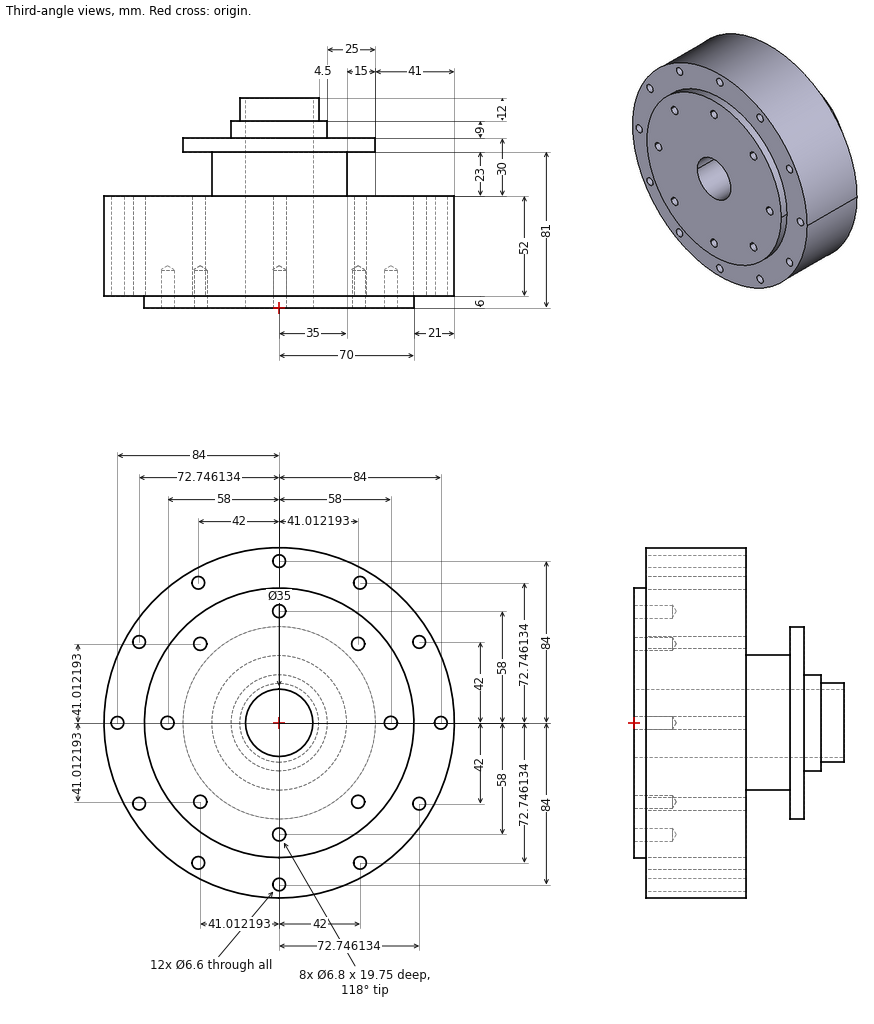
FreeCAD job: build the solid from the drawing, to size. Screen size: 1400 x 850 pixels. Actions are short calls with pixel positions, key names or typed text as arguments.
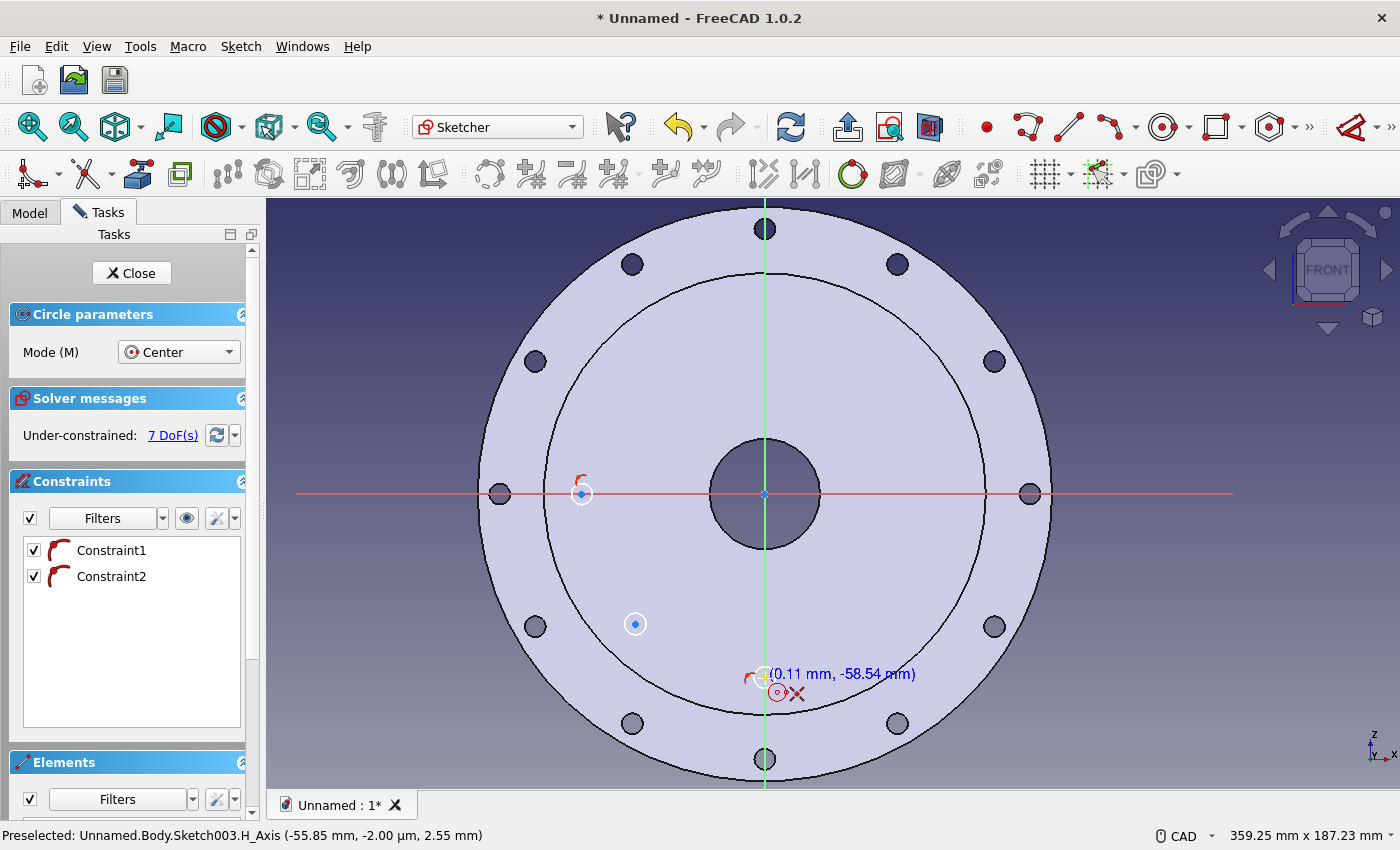
scroll(635, 365, up, 4)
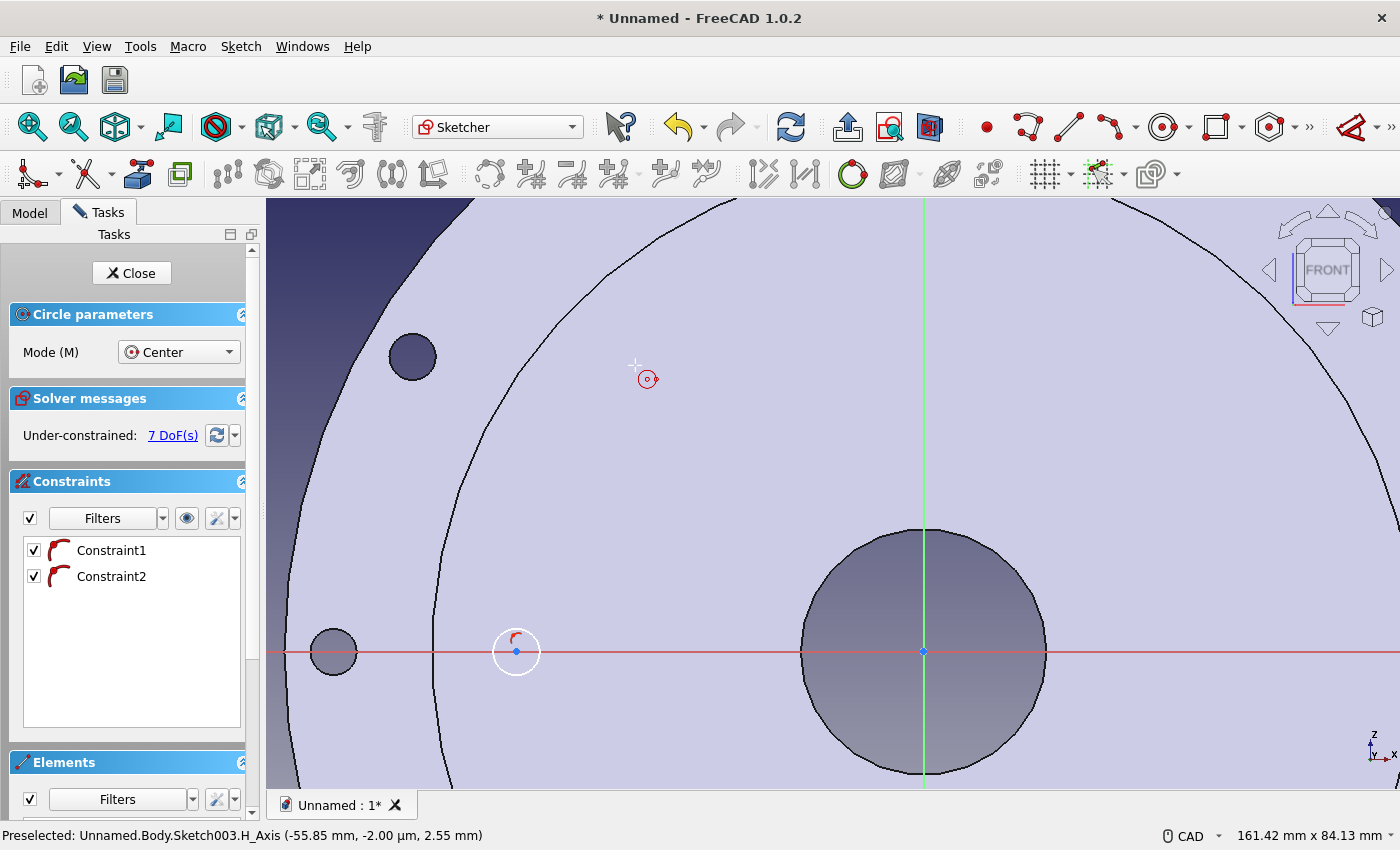
click(636, 364)
click(652, 347)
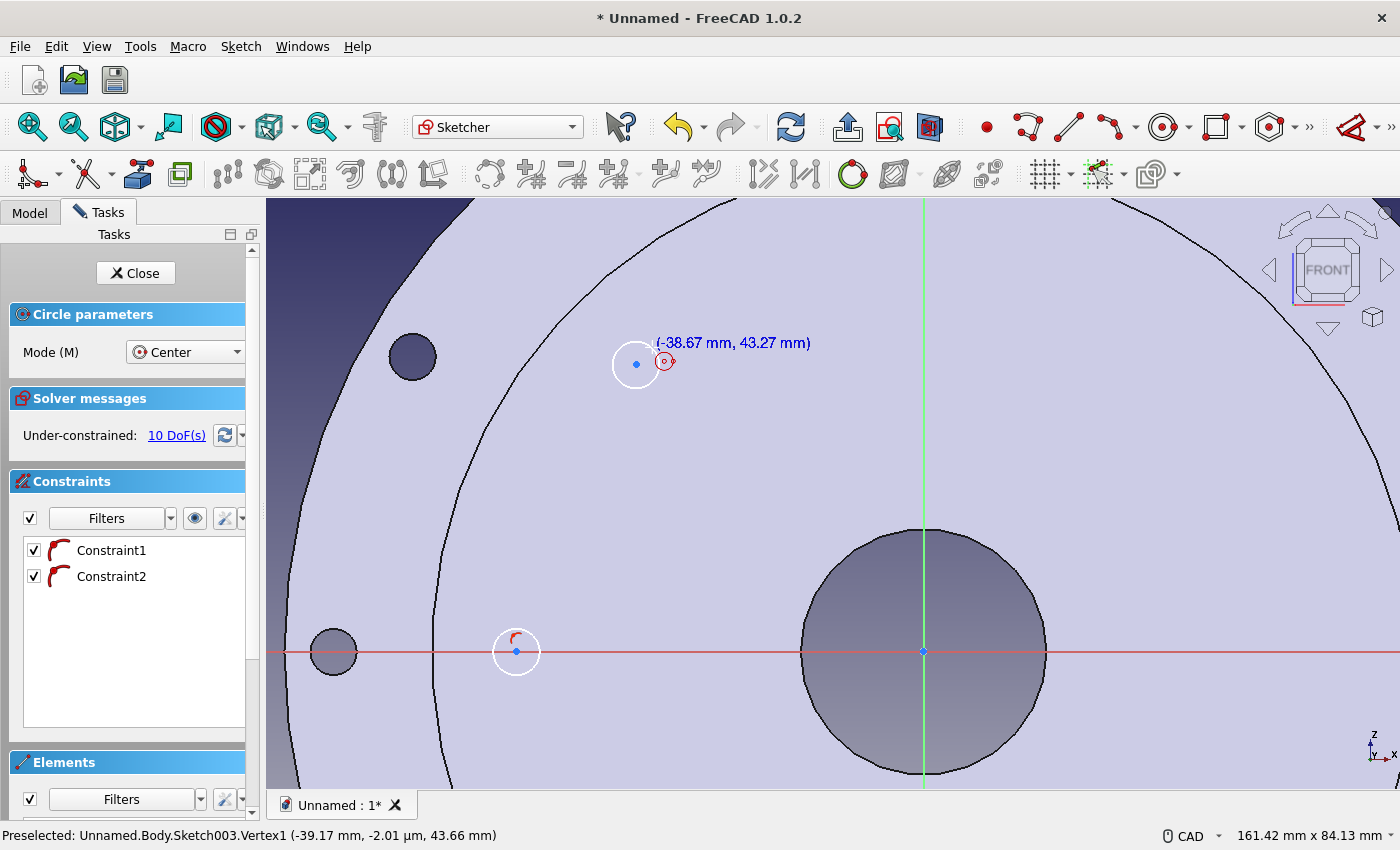
click(924, 245)
click(941, 228)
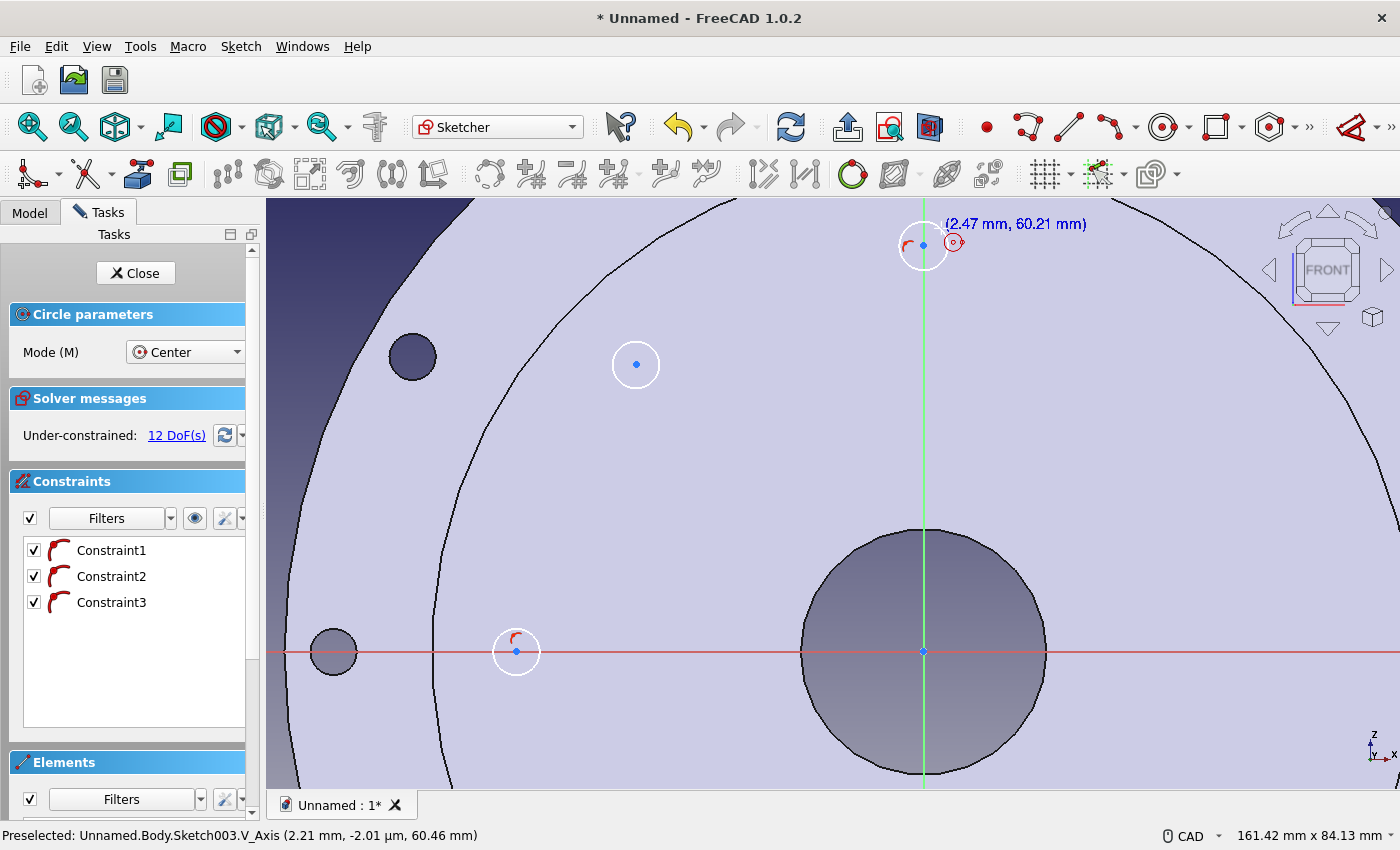
click(1212, 364)
click(1229, 347)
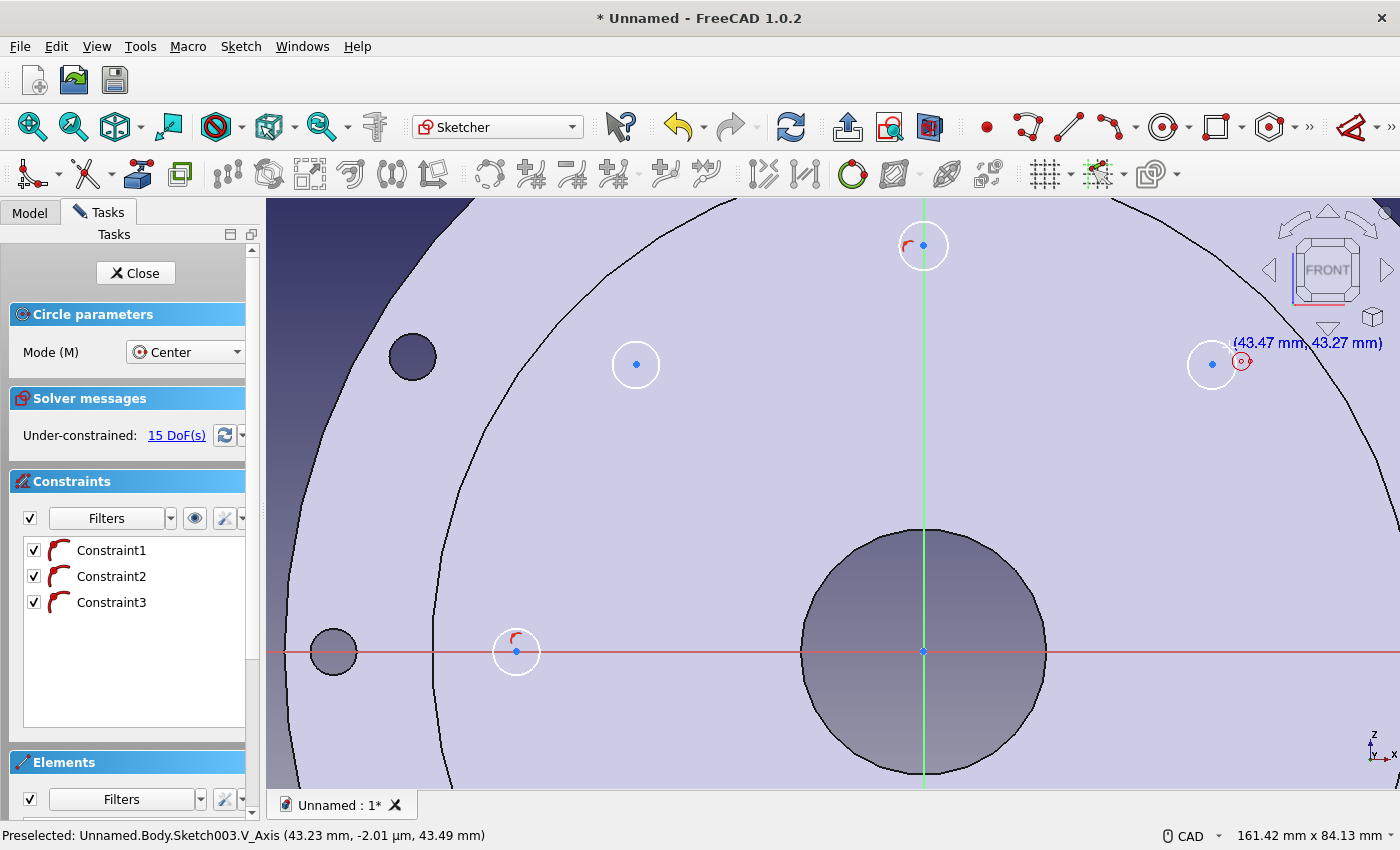
scroll(635, 364, down, 4)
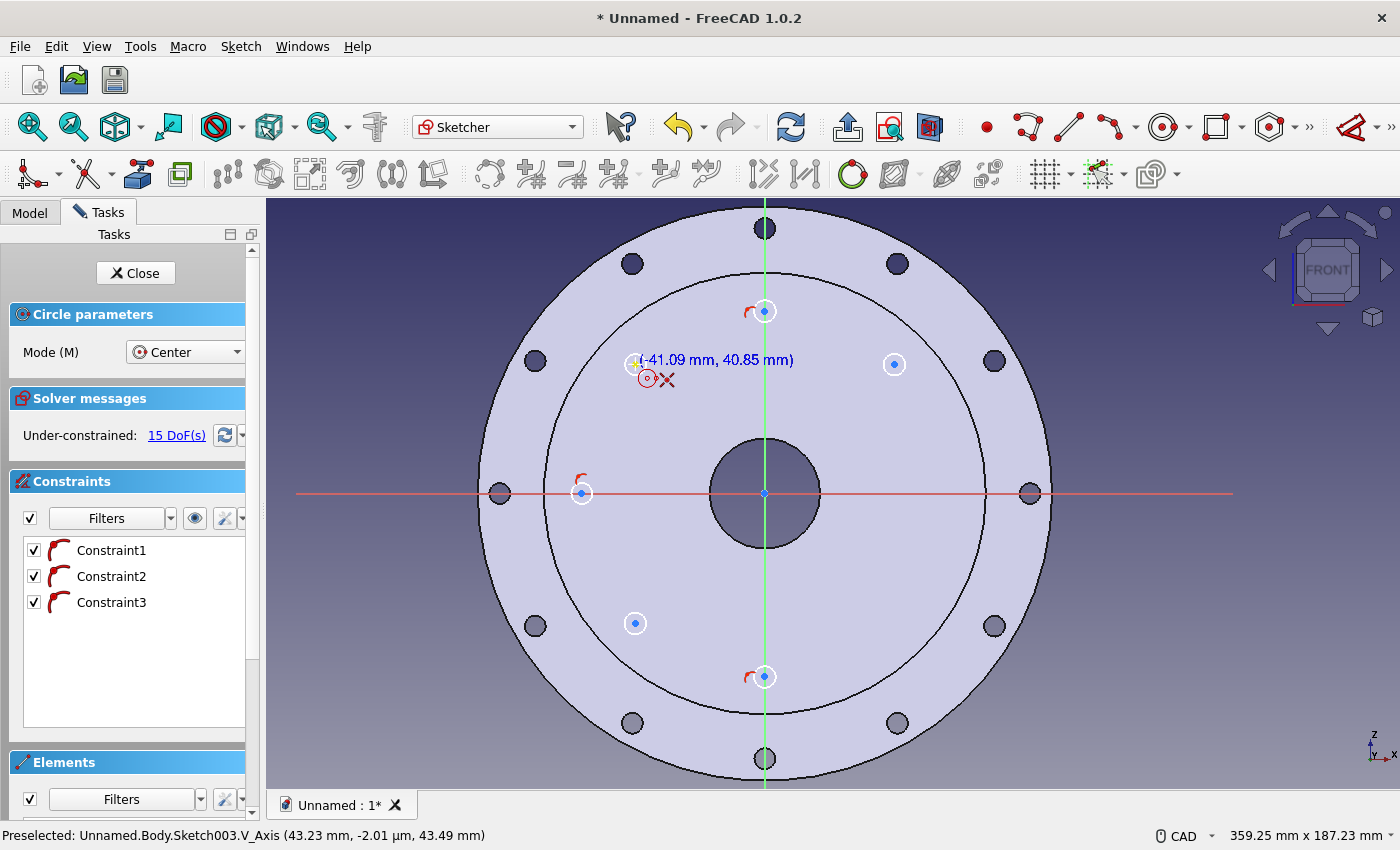
scroll(948, 494, up, 4)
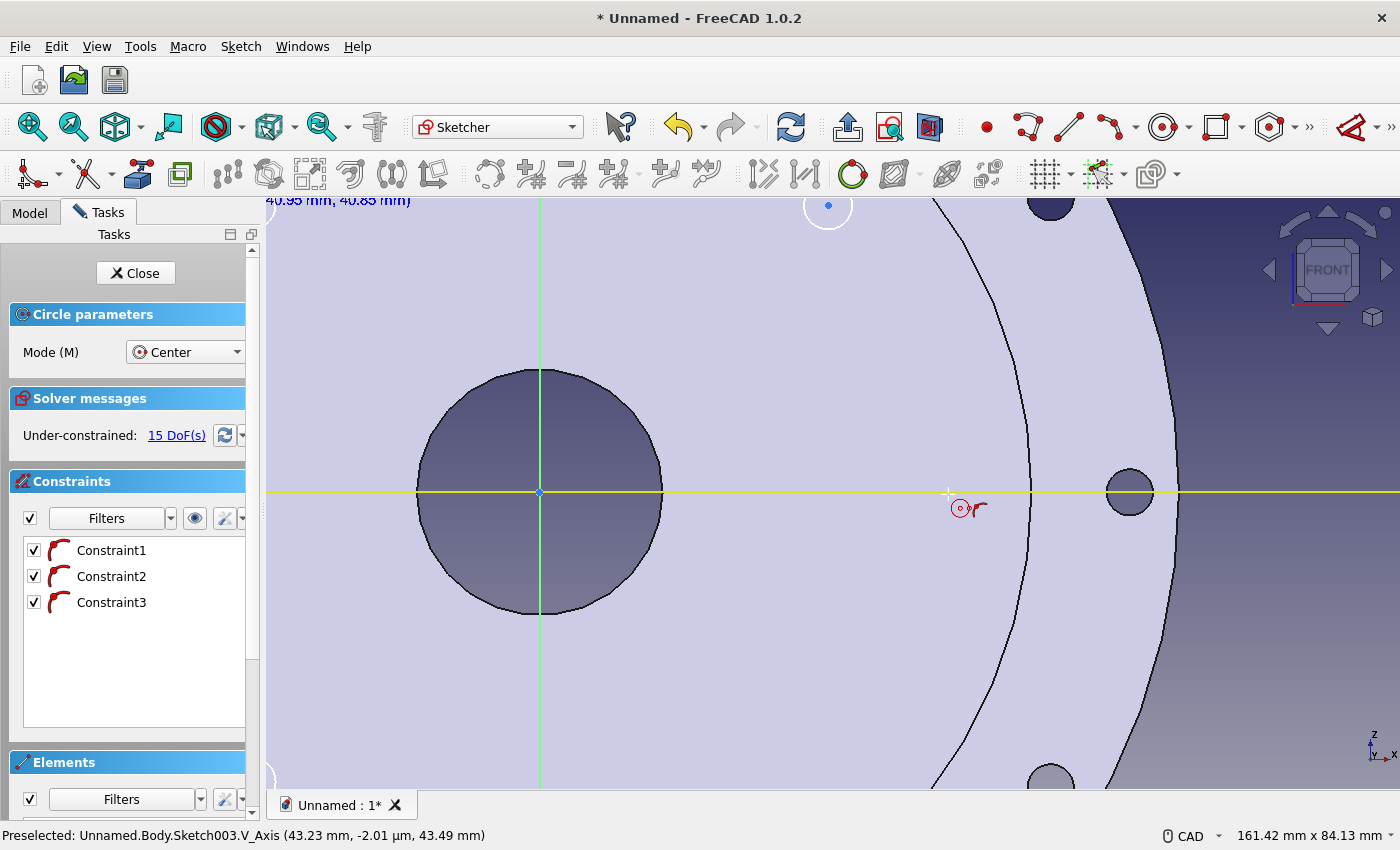
click(947, 492)
click(964, 476)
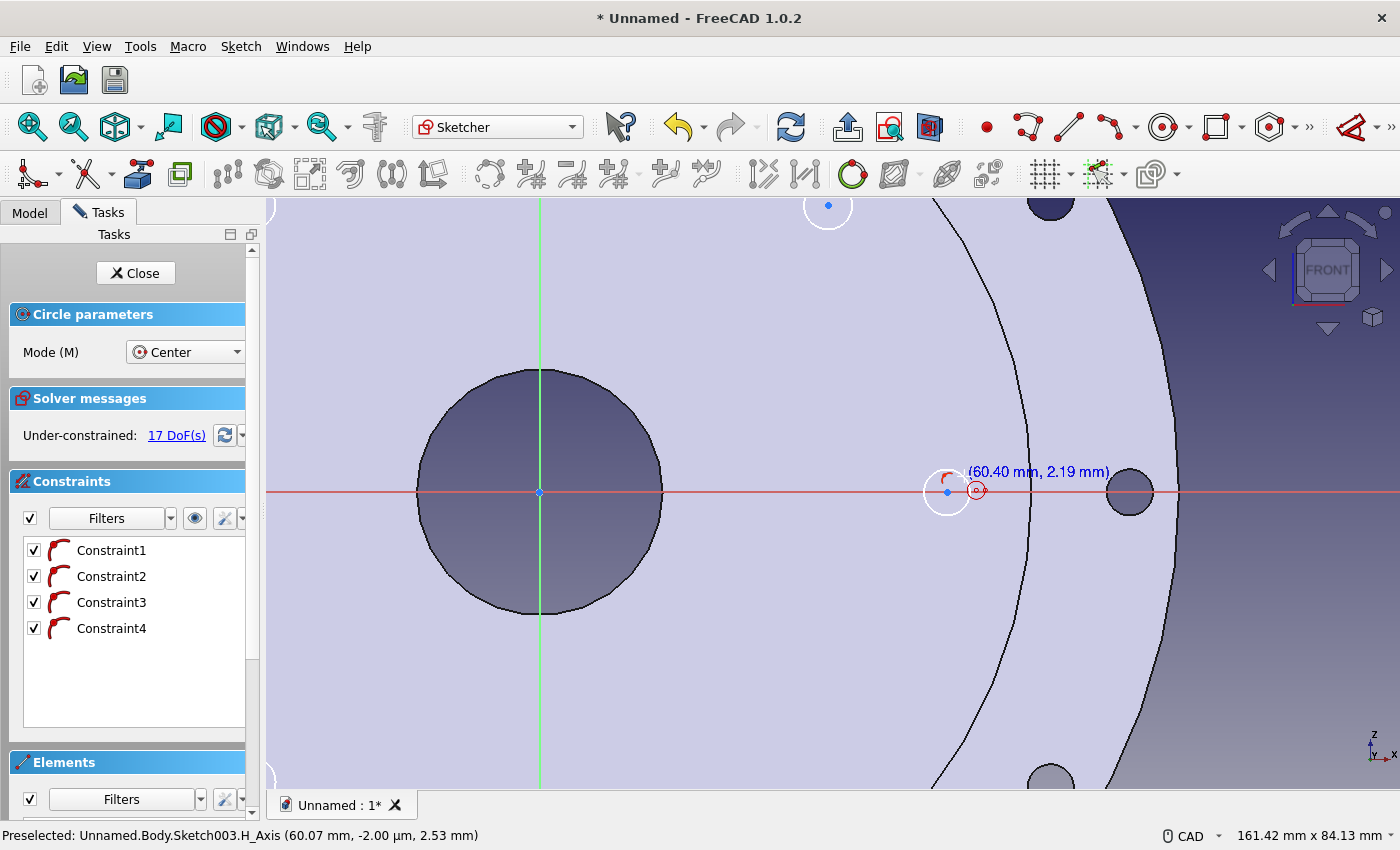
scroll(948, 494, down, 4)